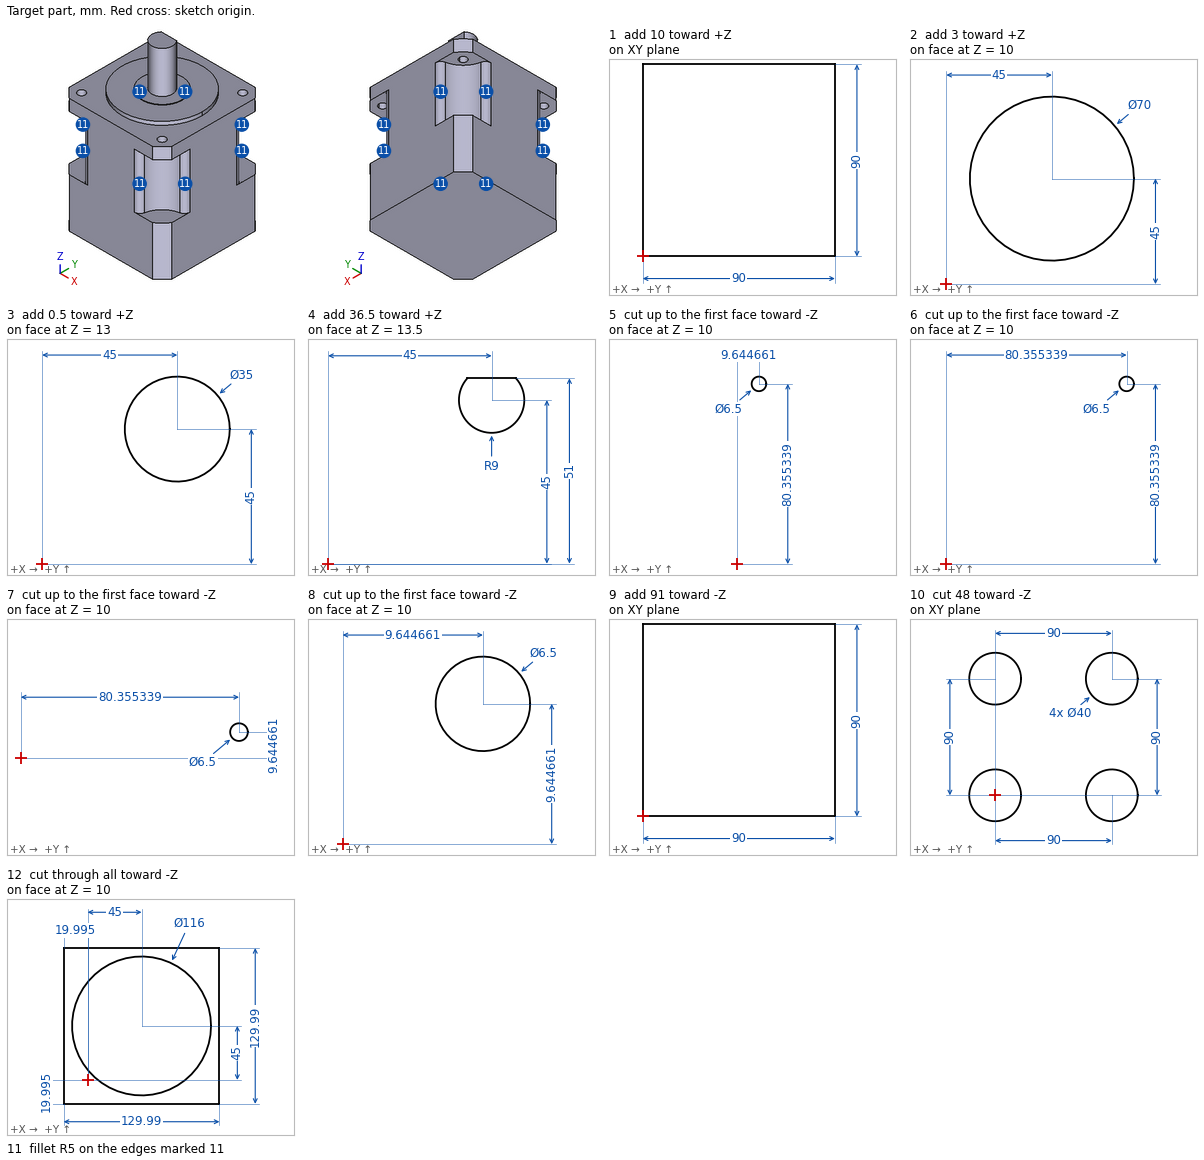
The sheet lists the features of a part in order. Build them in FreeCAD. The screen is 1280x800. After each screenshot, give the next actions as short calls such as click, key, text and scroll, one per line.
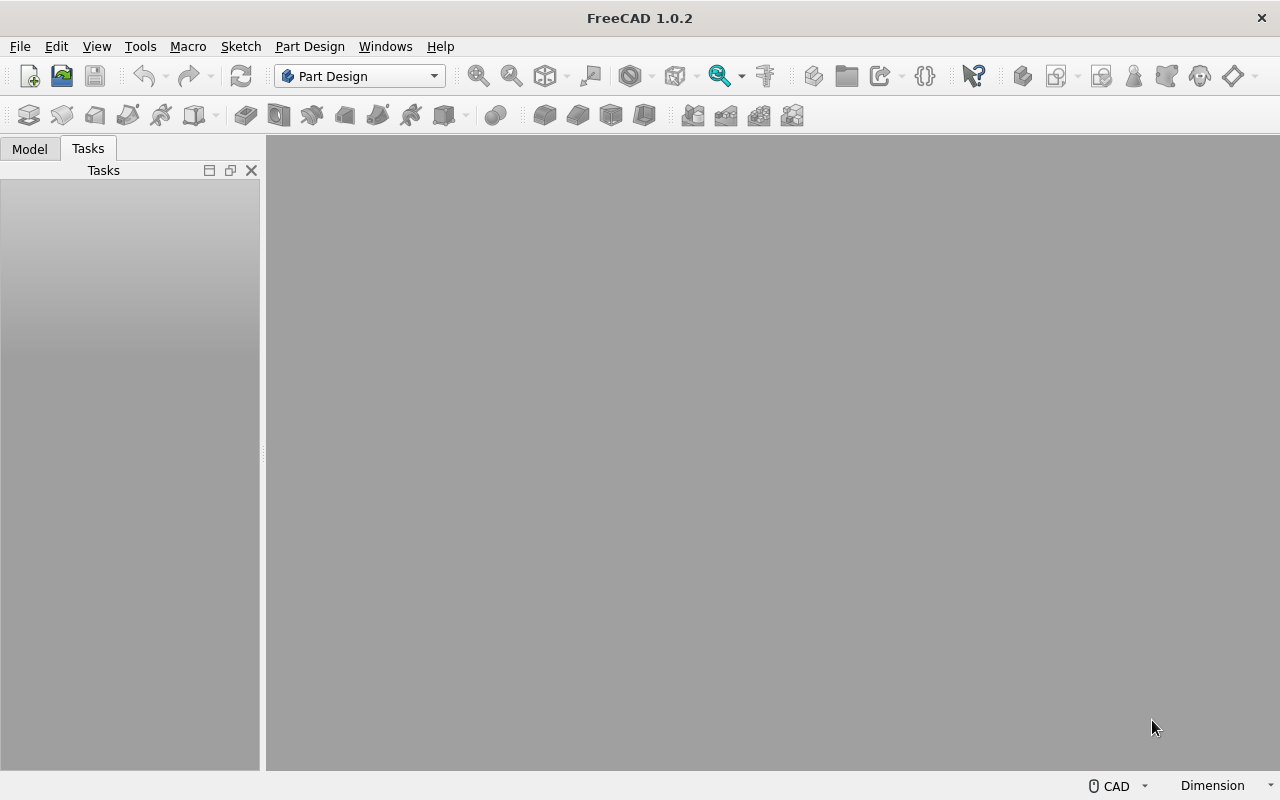
key(ctrl+n)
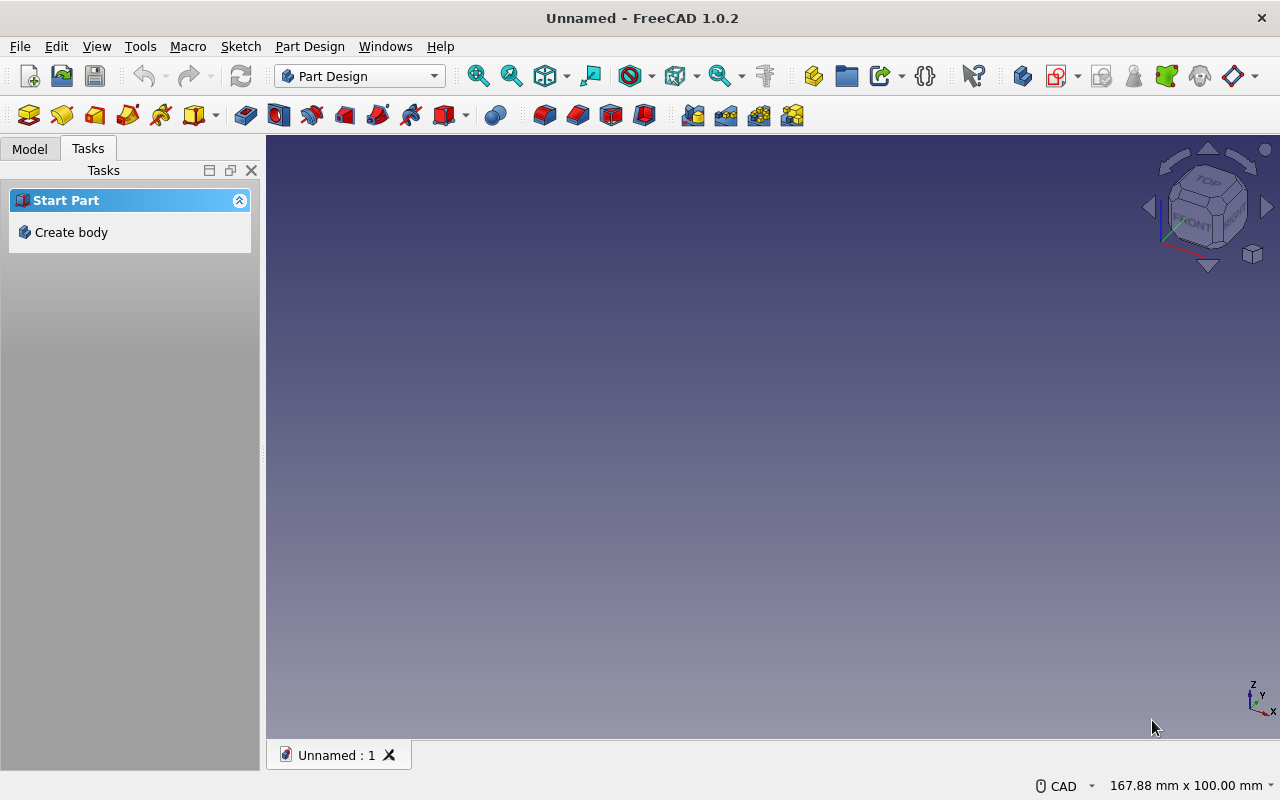
click(1056, 76)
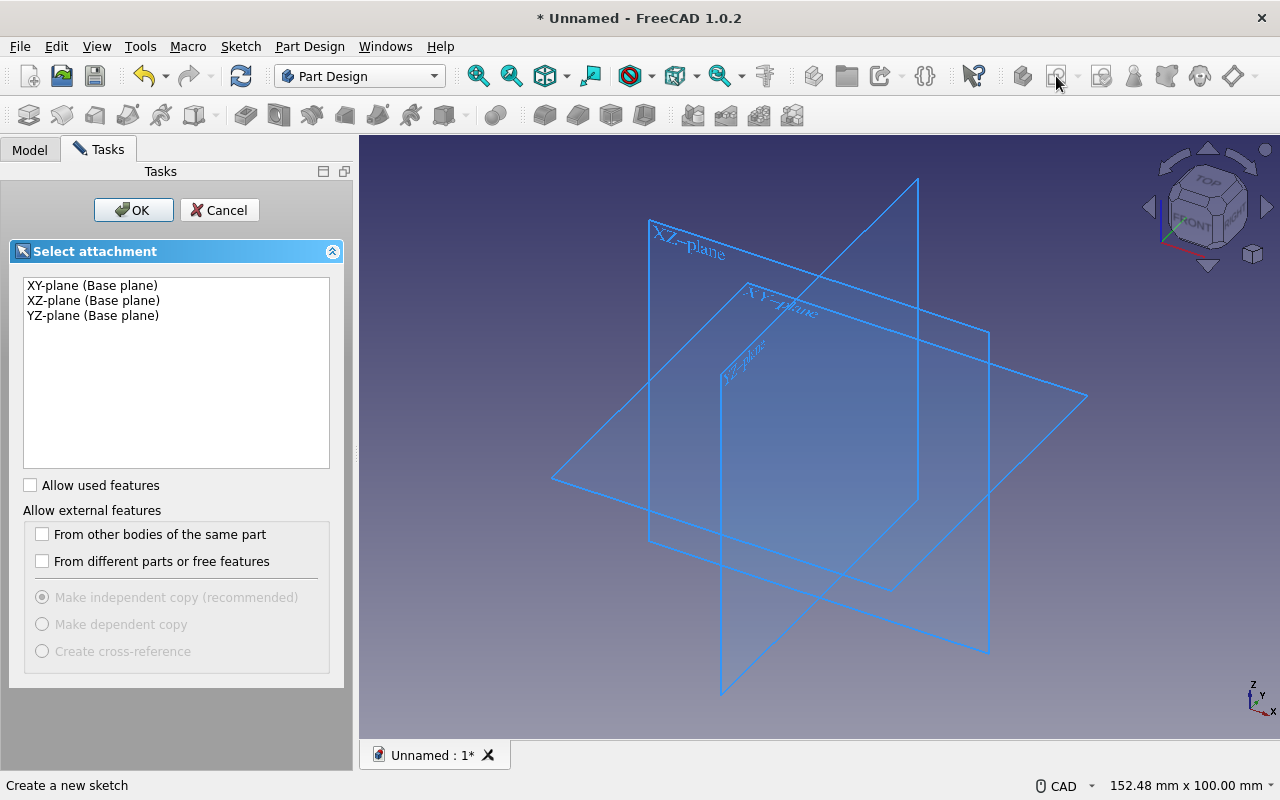
click(84, 286)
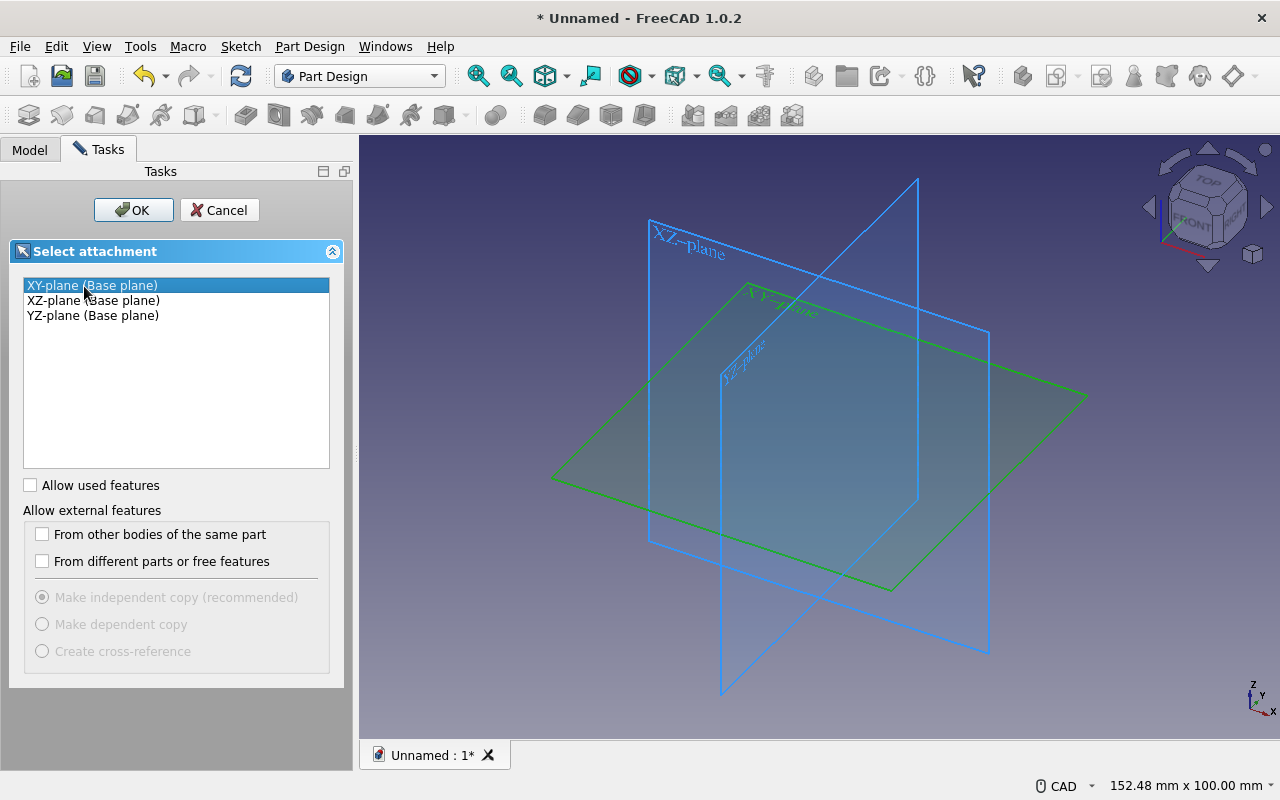
click(134, 210)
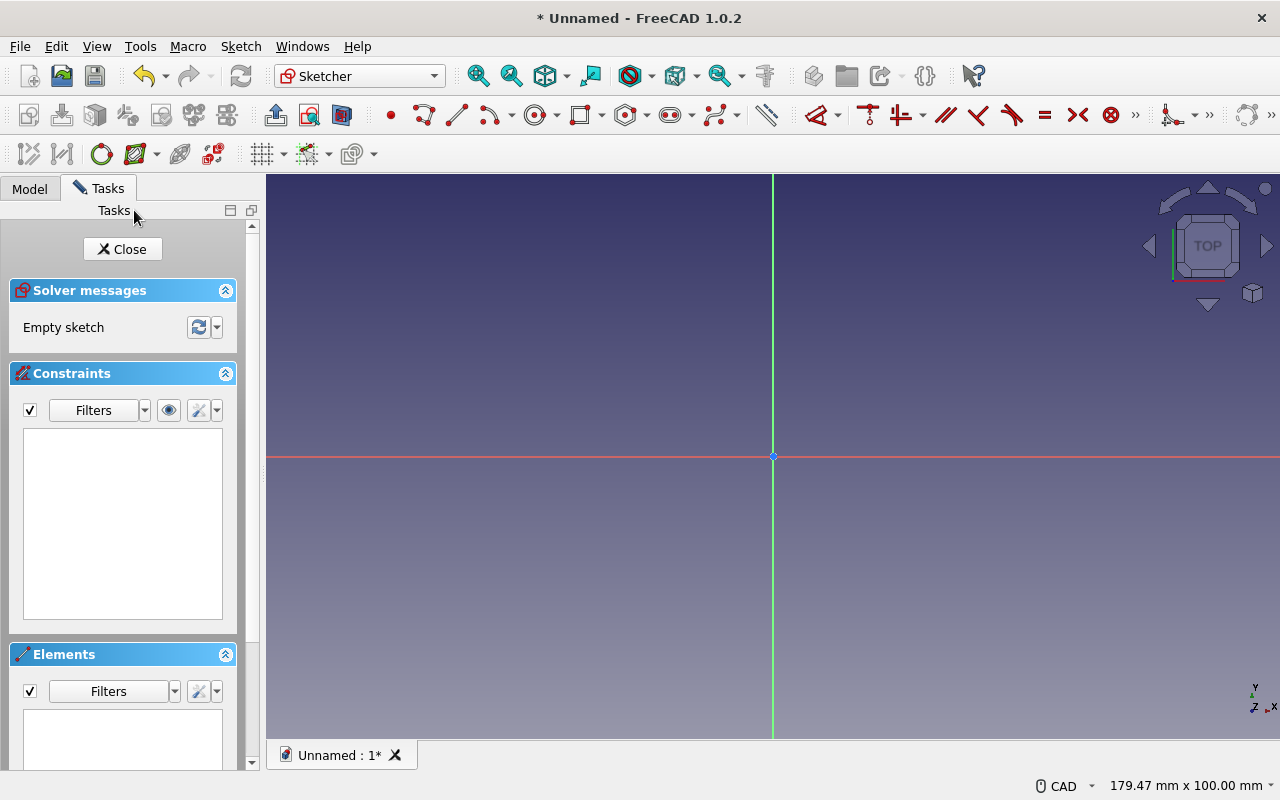
scroll(312, 711, down, 3)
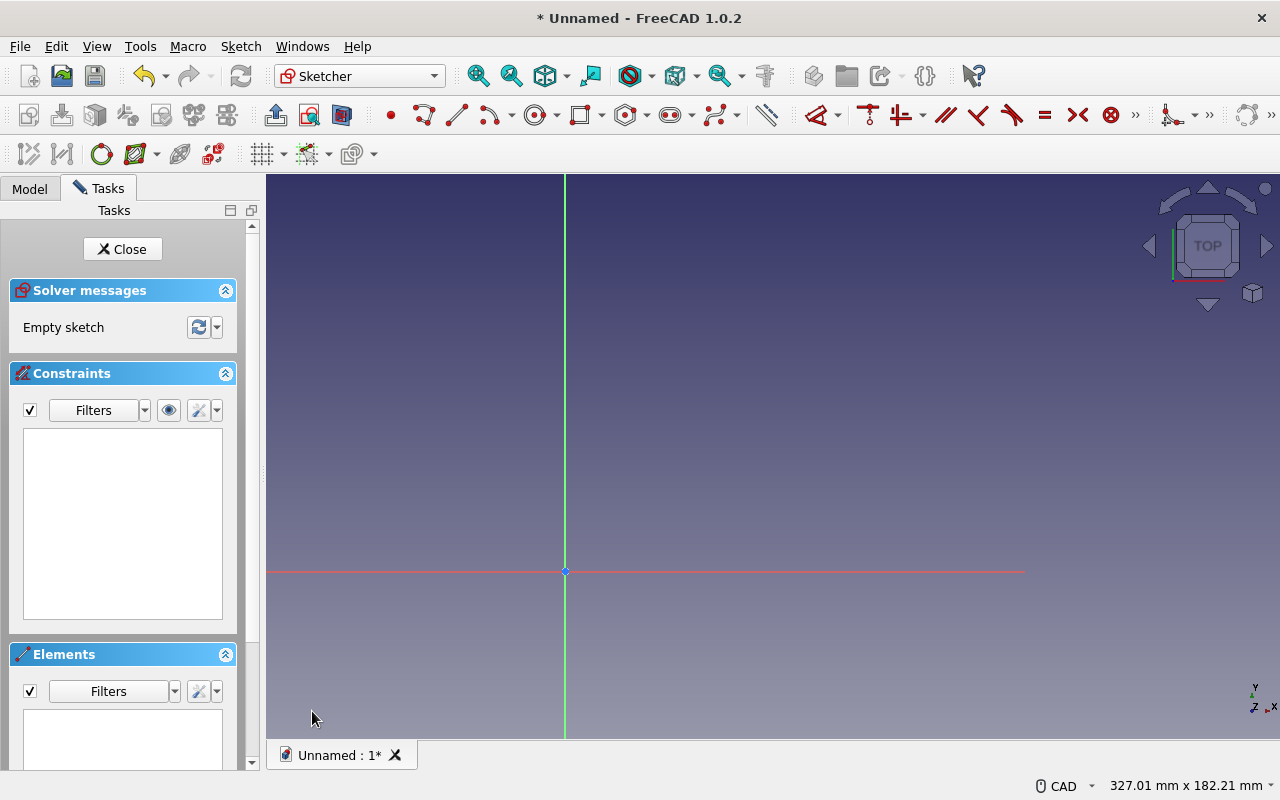
key(g)
key(r)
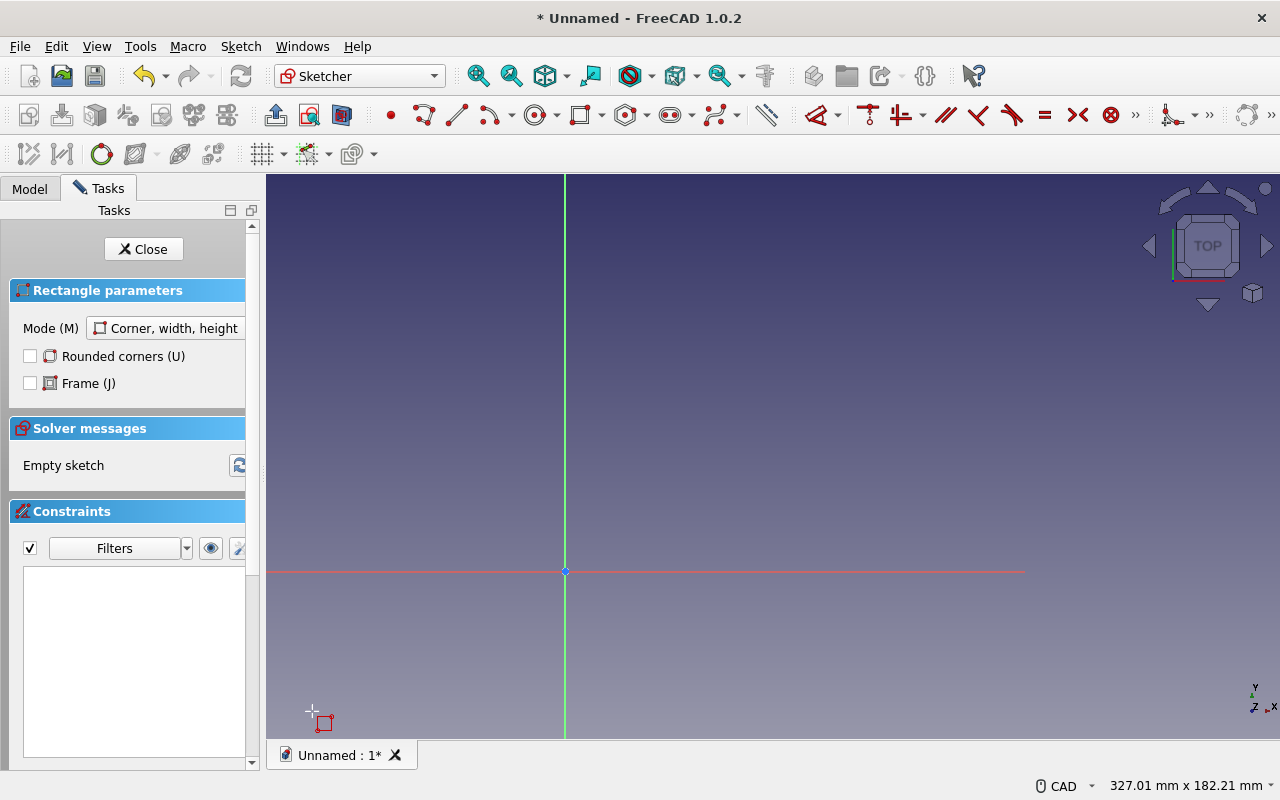
click(565, 572)
move(844, 293)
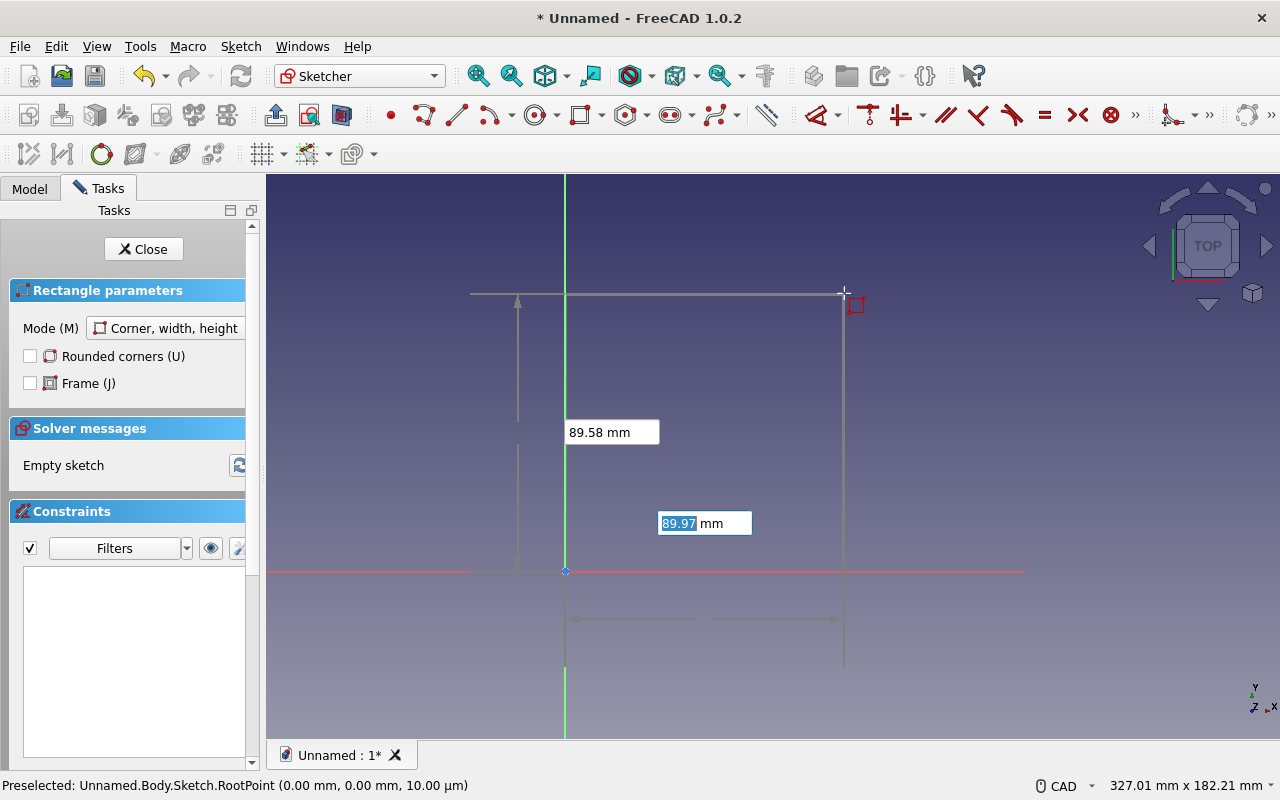
text(90)
key(Tab)
text(90)
key(Return)
key(Escape)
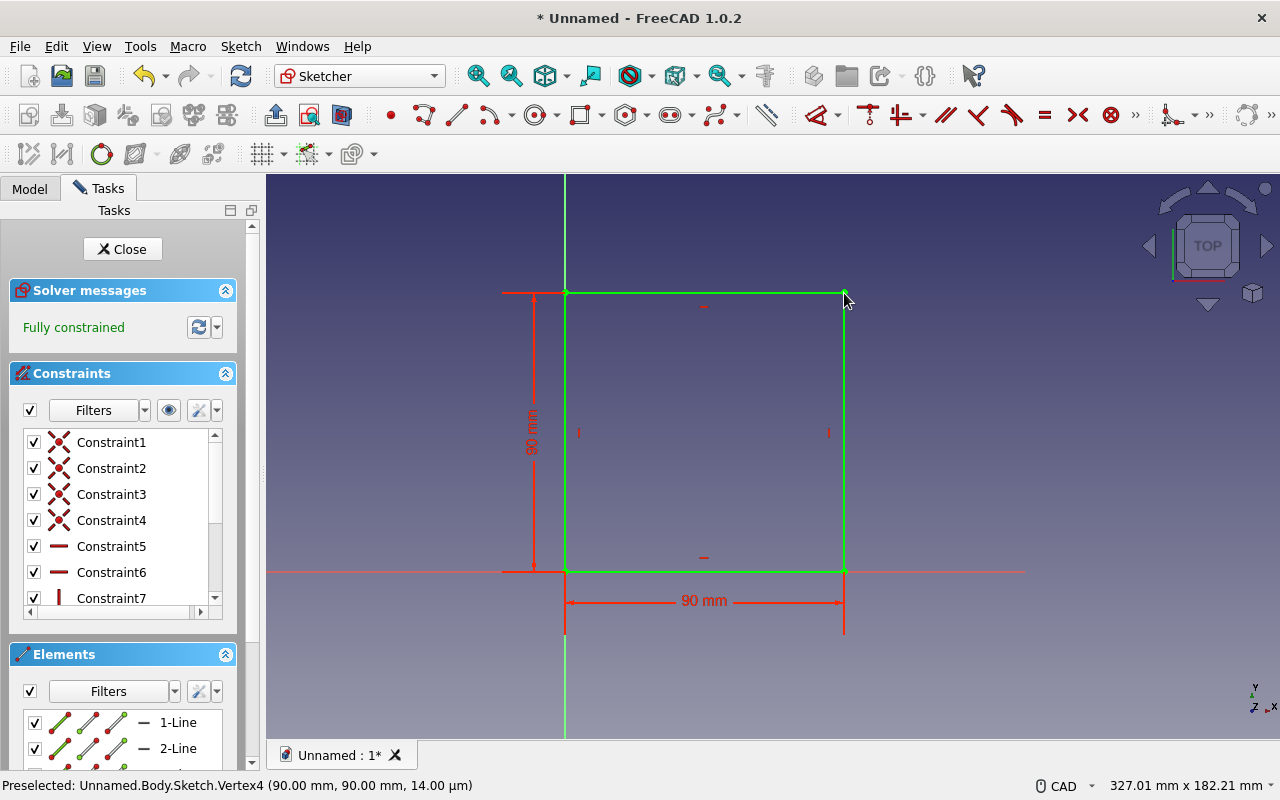
click(123, 249)